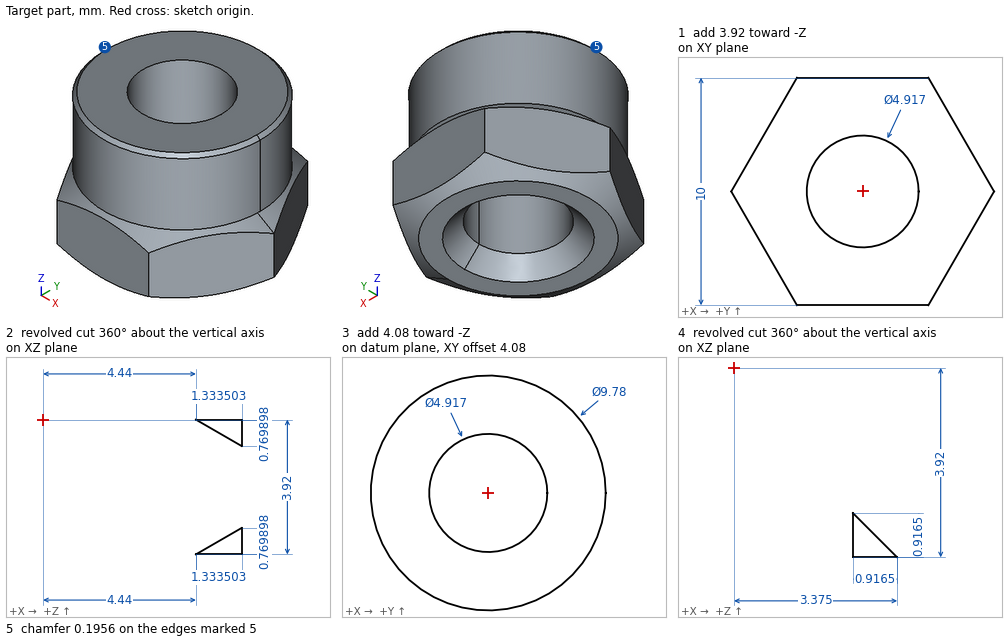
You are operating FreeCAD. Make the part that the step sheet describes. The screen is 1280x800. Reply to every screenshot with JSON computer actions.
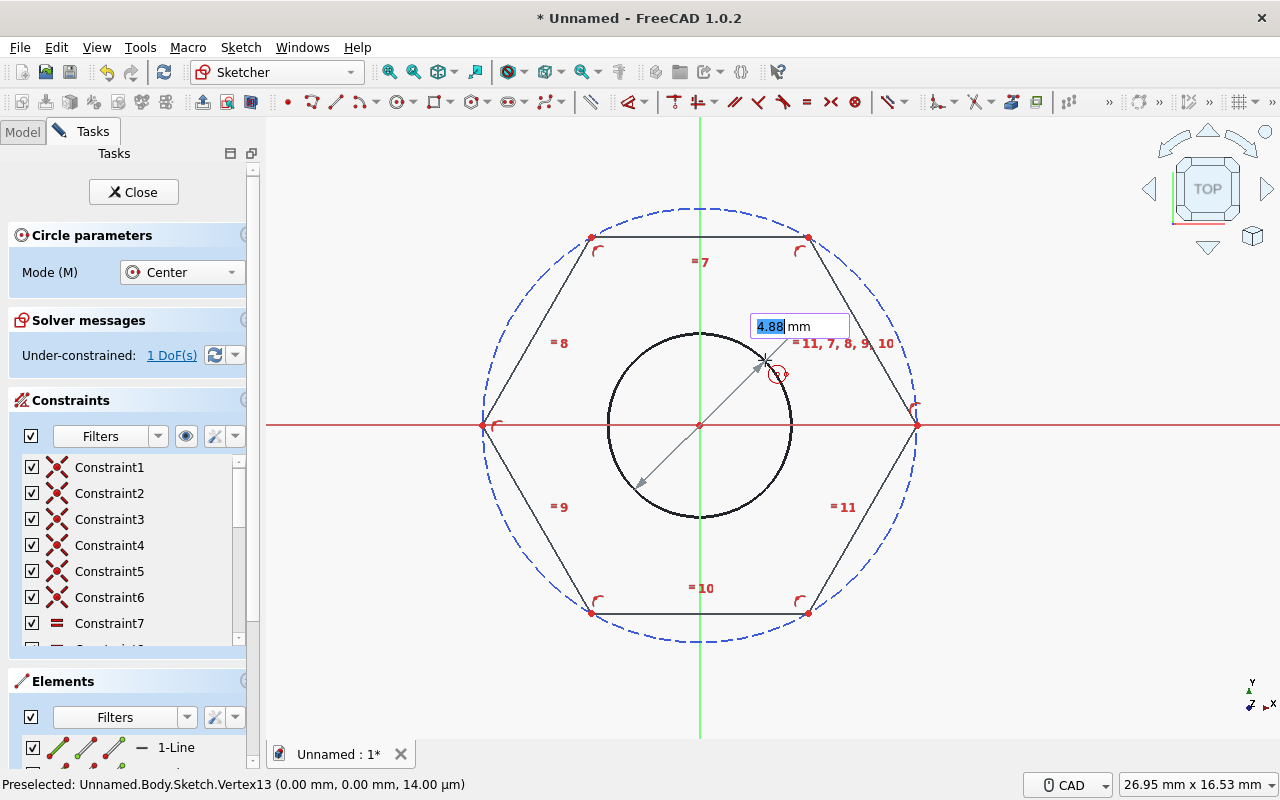
{"action": "type", "text": "4.917"}
{"action": "key", "text": "Return"}
{"action": "key", "text": "Escape"}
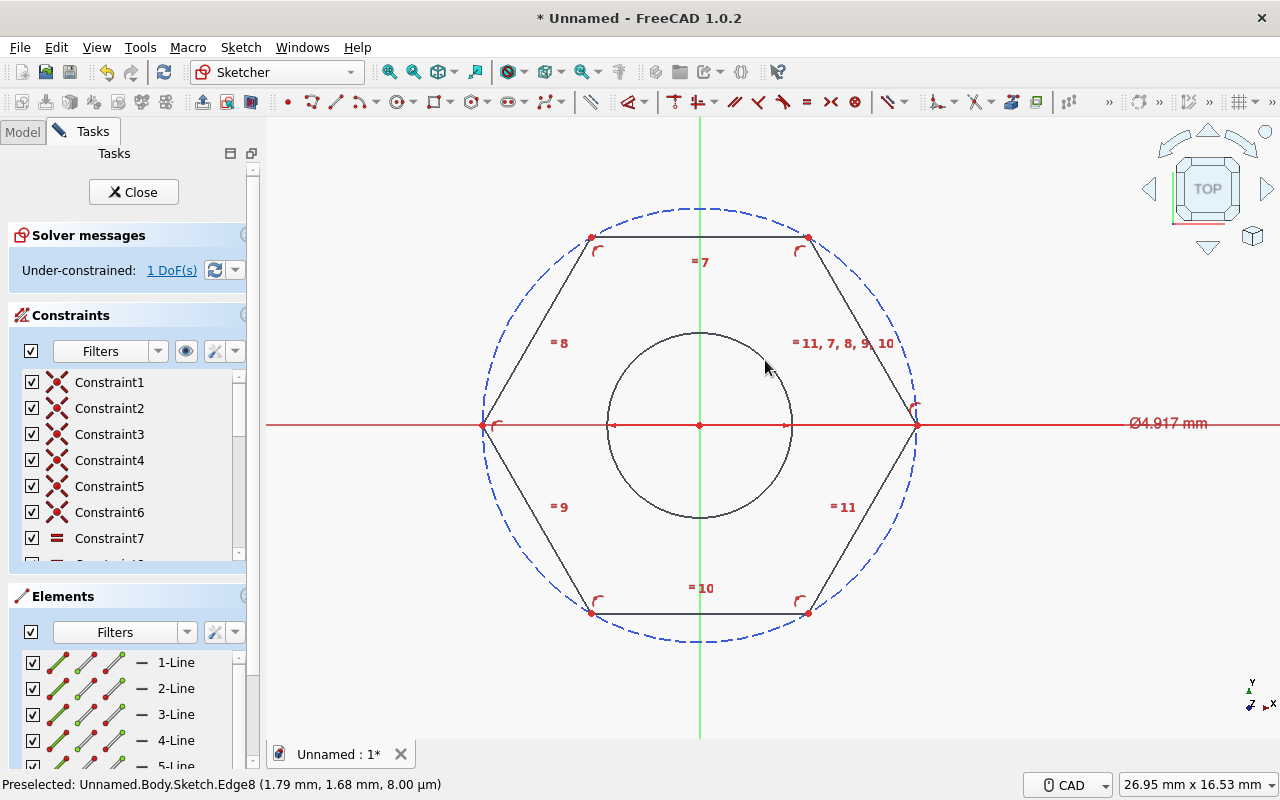
{"action": "left_click", "coordinate": [628, 102]}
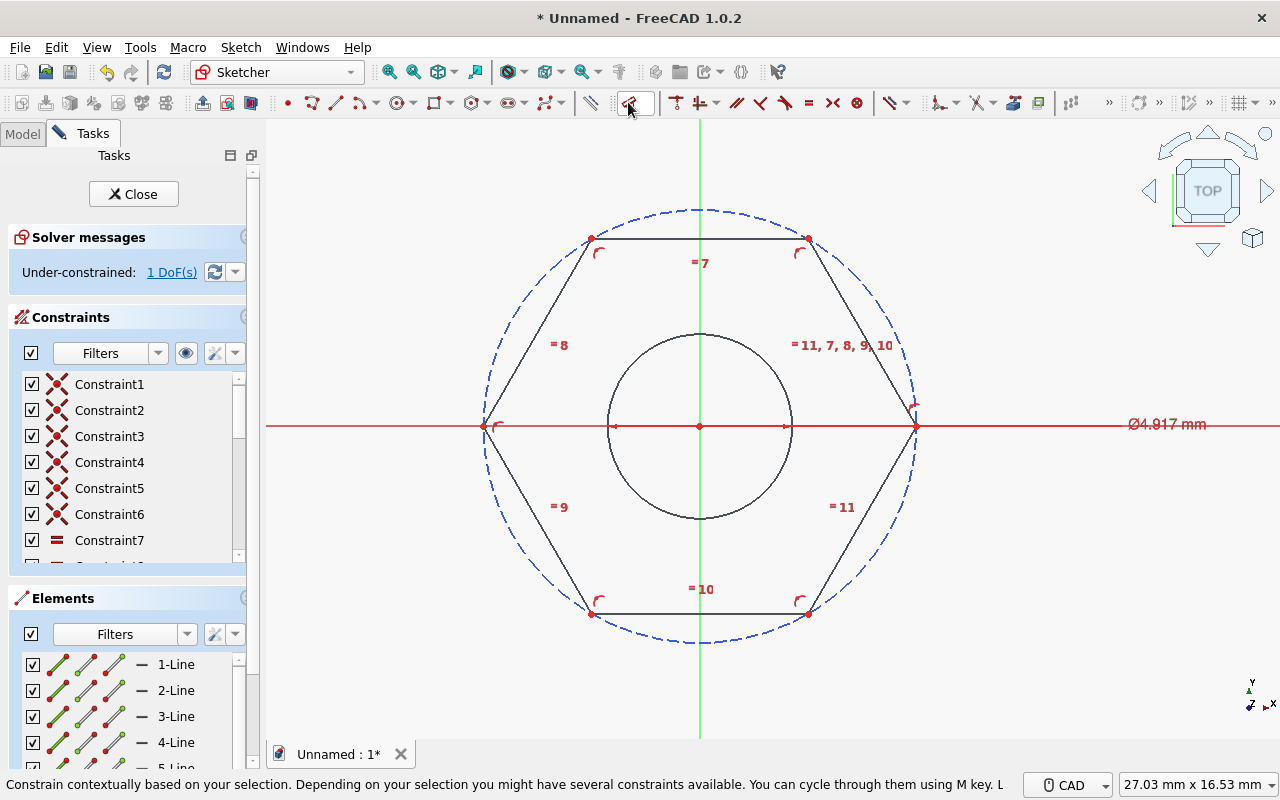
{"action": "left_click", "coordinate": [592, 614]}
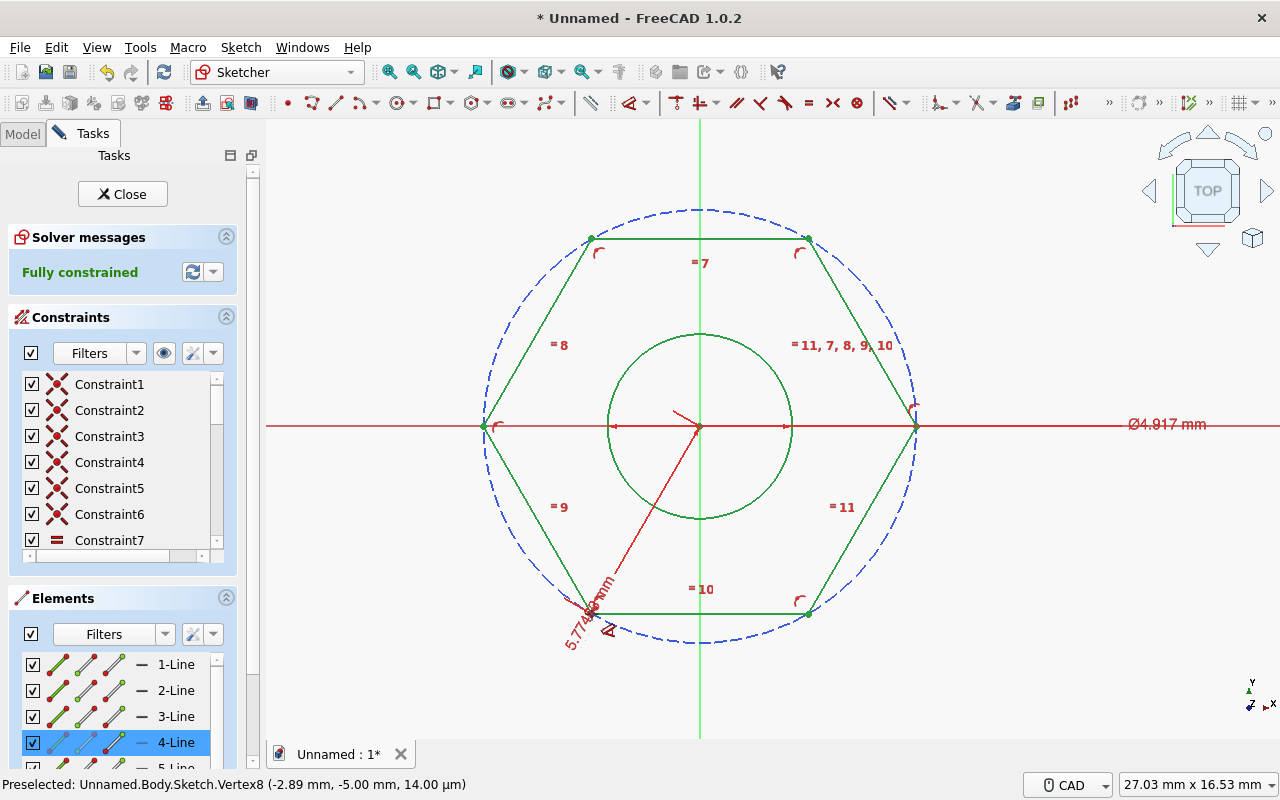
{"action": "left_click", "coordinate": [808, 239]}
{"action": "left_click", "coordinate": [558, 340]}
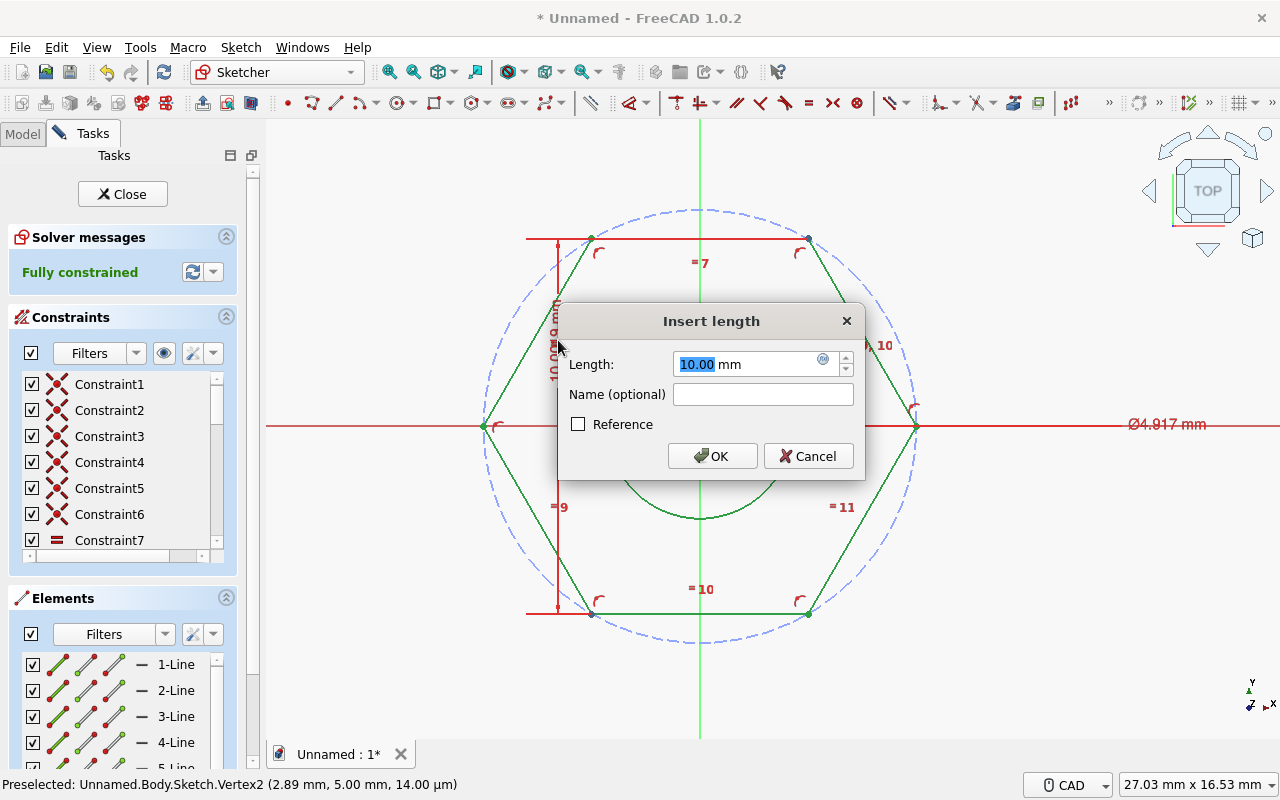
{"action": "type", "text": "10"}
{"action": "key", "text": "Return"}
{"action": "key", "text": "Escape"}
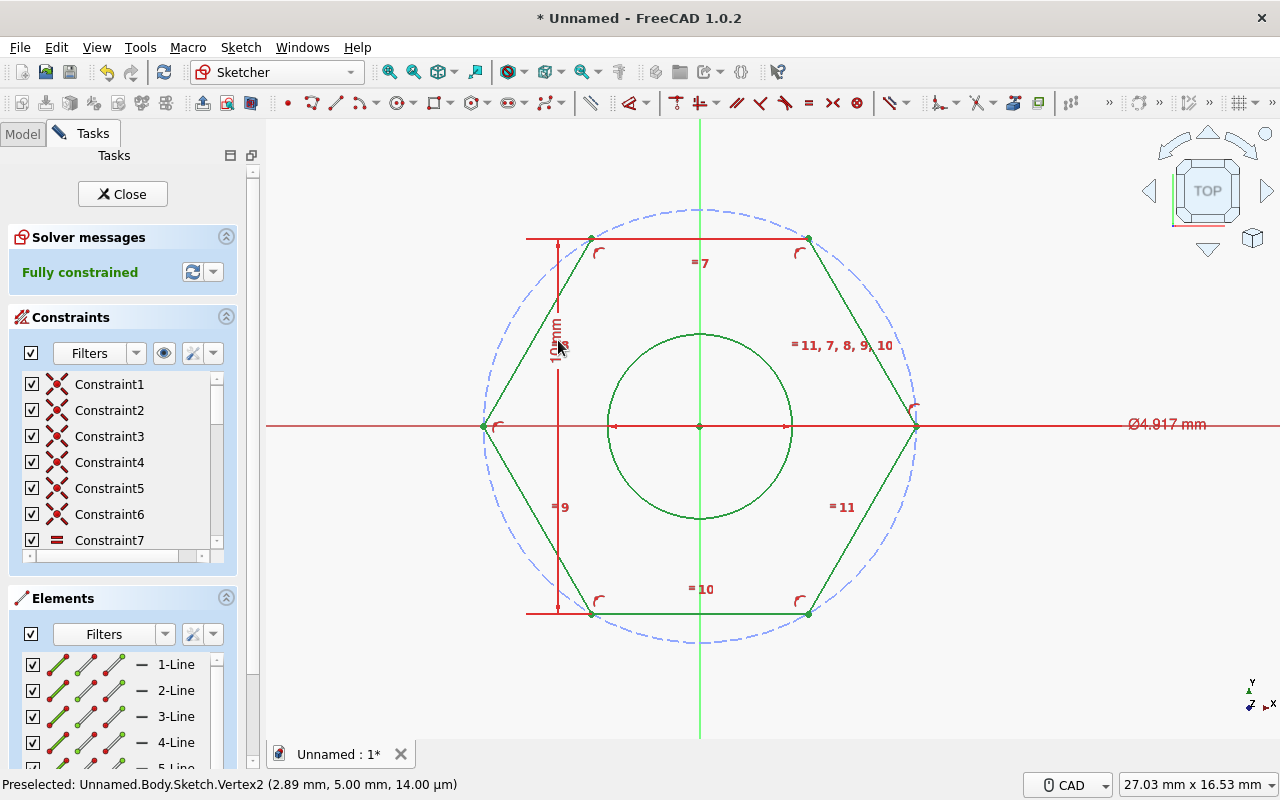
{"action": "left_click", "coordinate": [123, 194]}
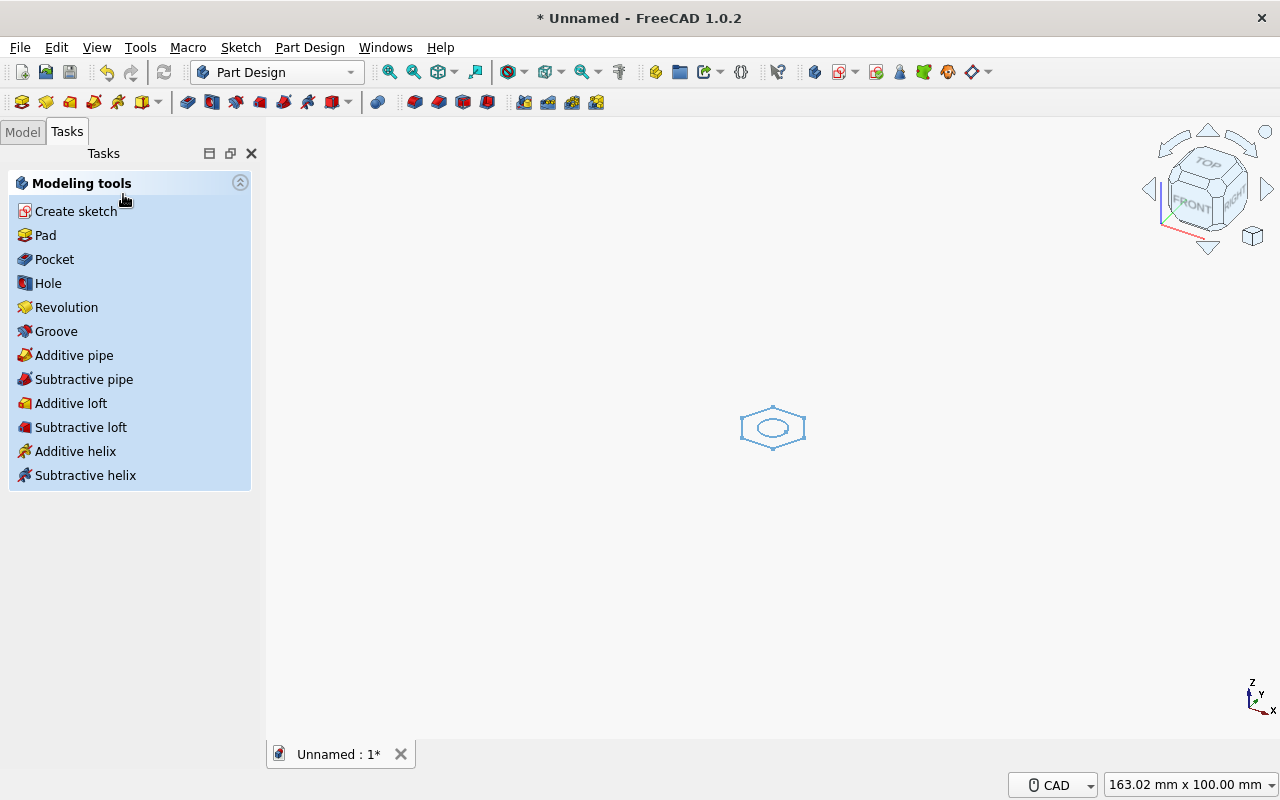
{"action": "left_click", "coordinate": [22, 102]}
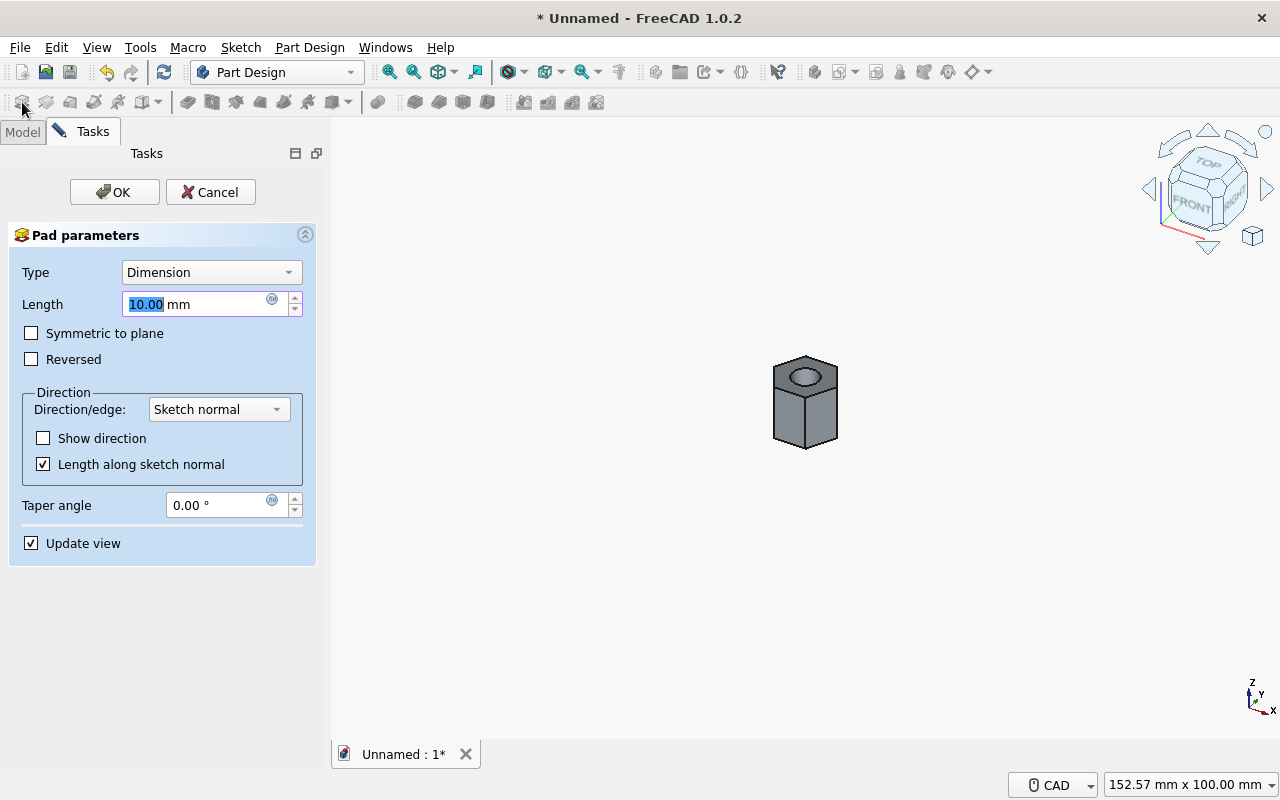
{"action": "type", "text": "3.92"}
{"action": "key", "text": "Tab"}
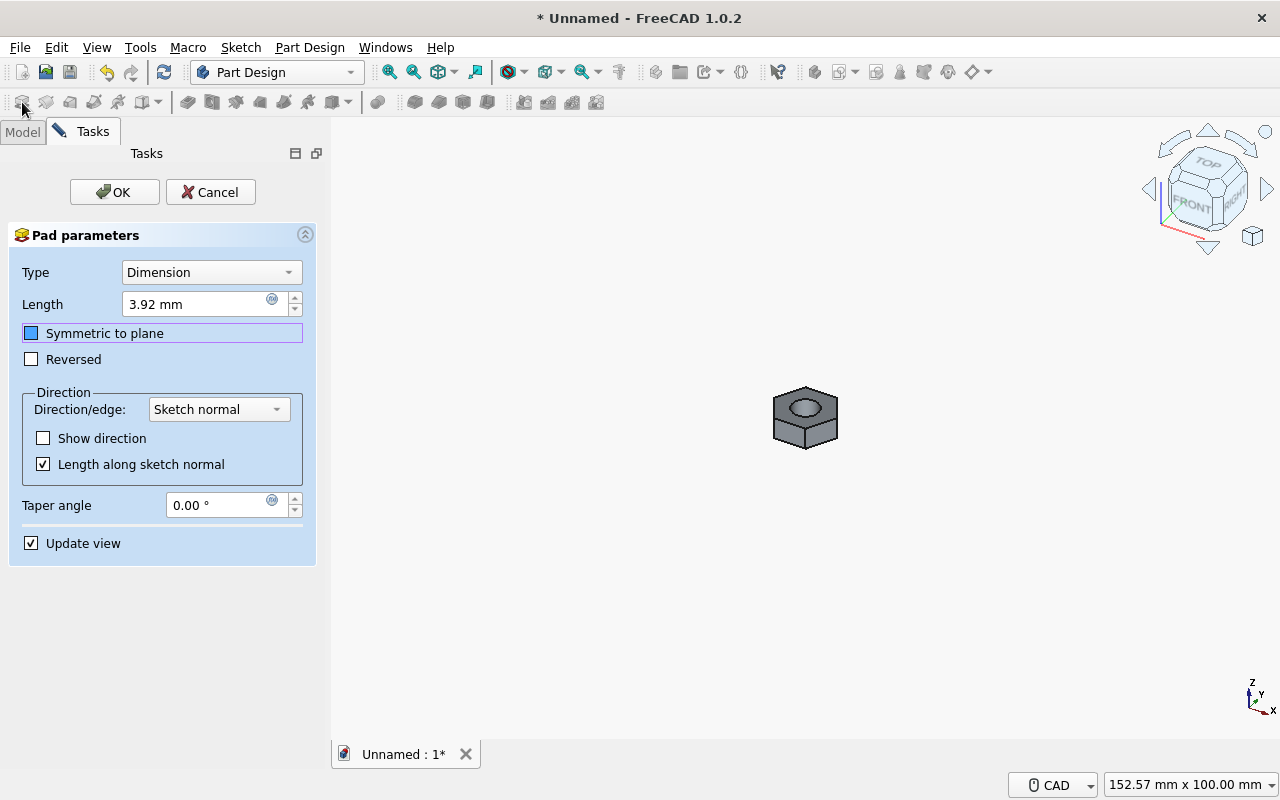
{"action": "left_click", "coordinate": [30, 359]}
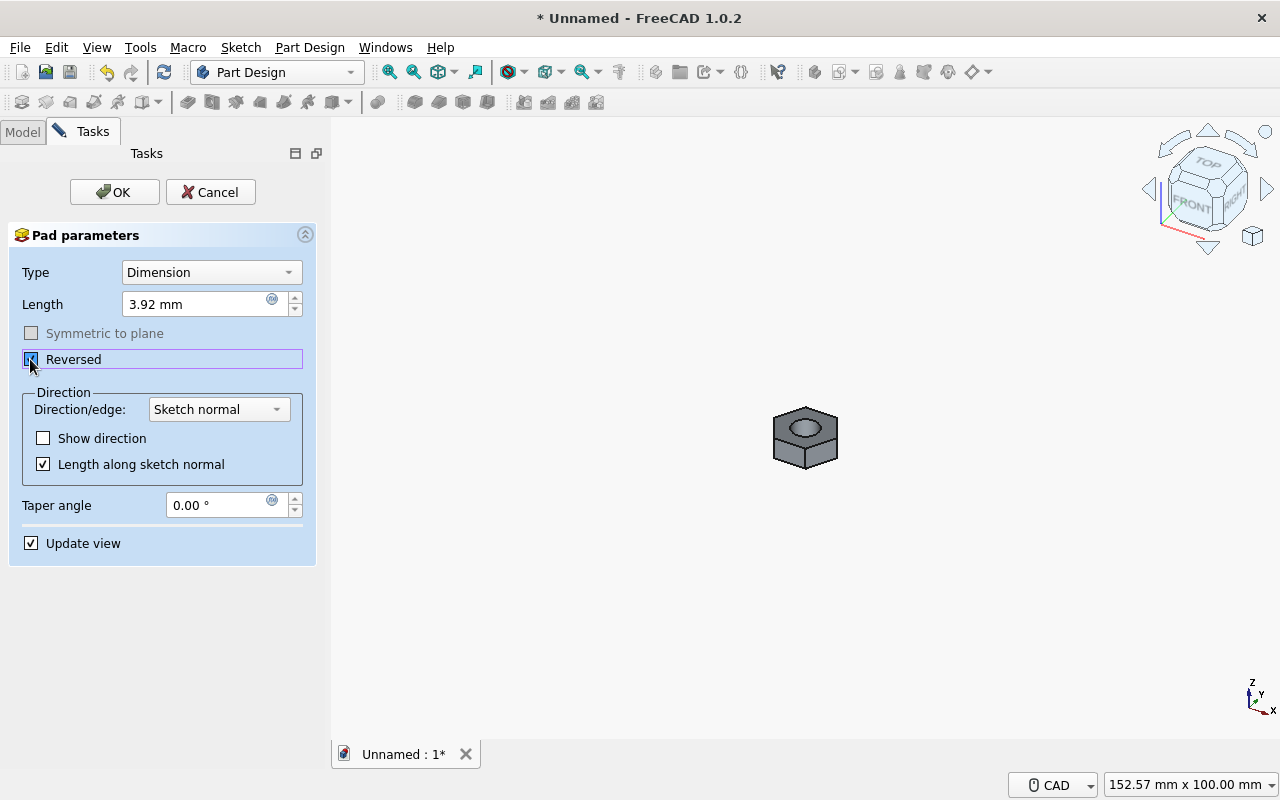
{"action": "left_click", "coordinate": [115, 192]}